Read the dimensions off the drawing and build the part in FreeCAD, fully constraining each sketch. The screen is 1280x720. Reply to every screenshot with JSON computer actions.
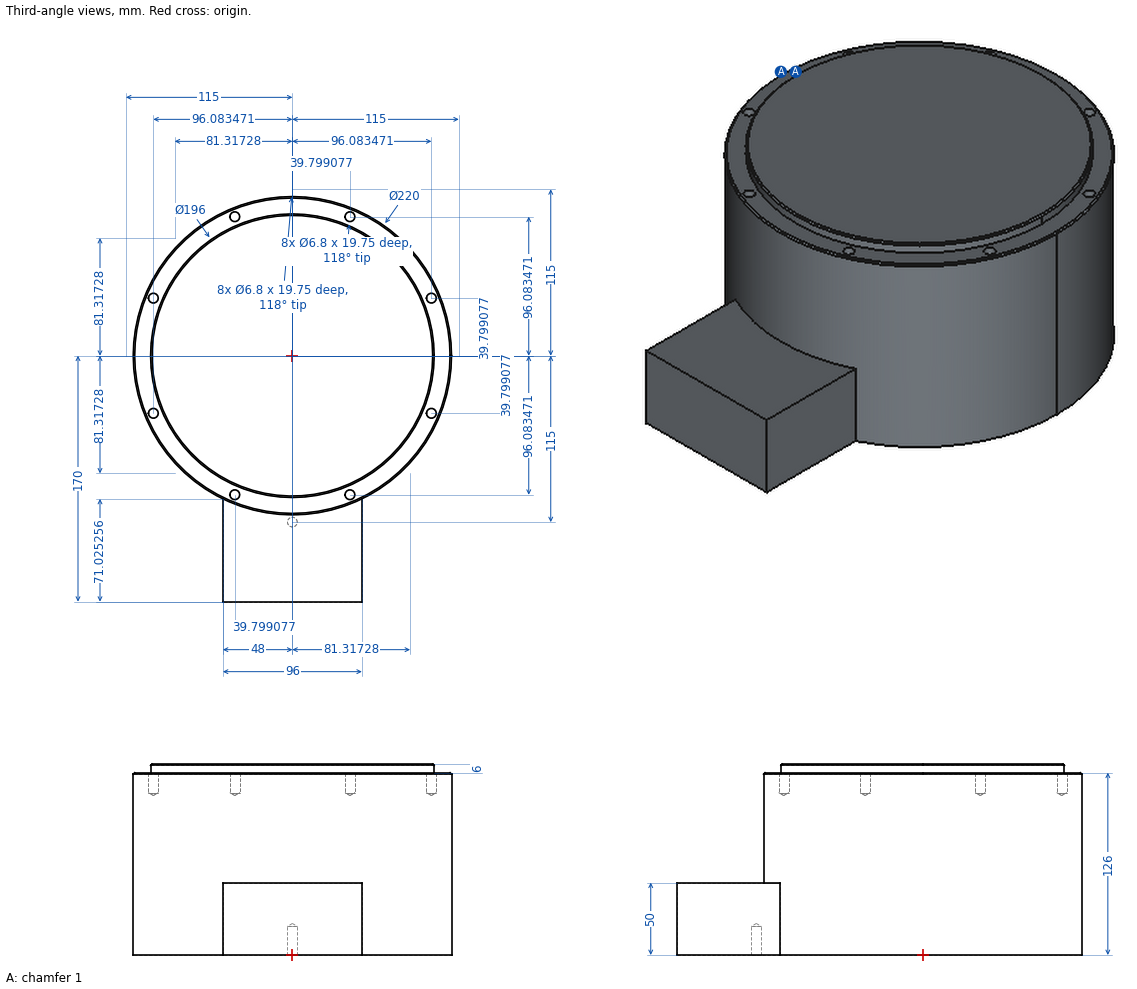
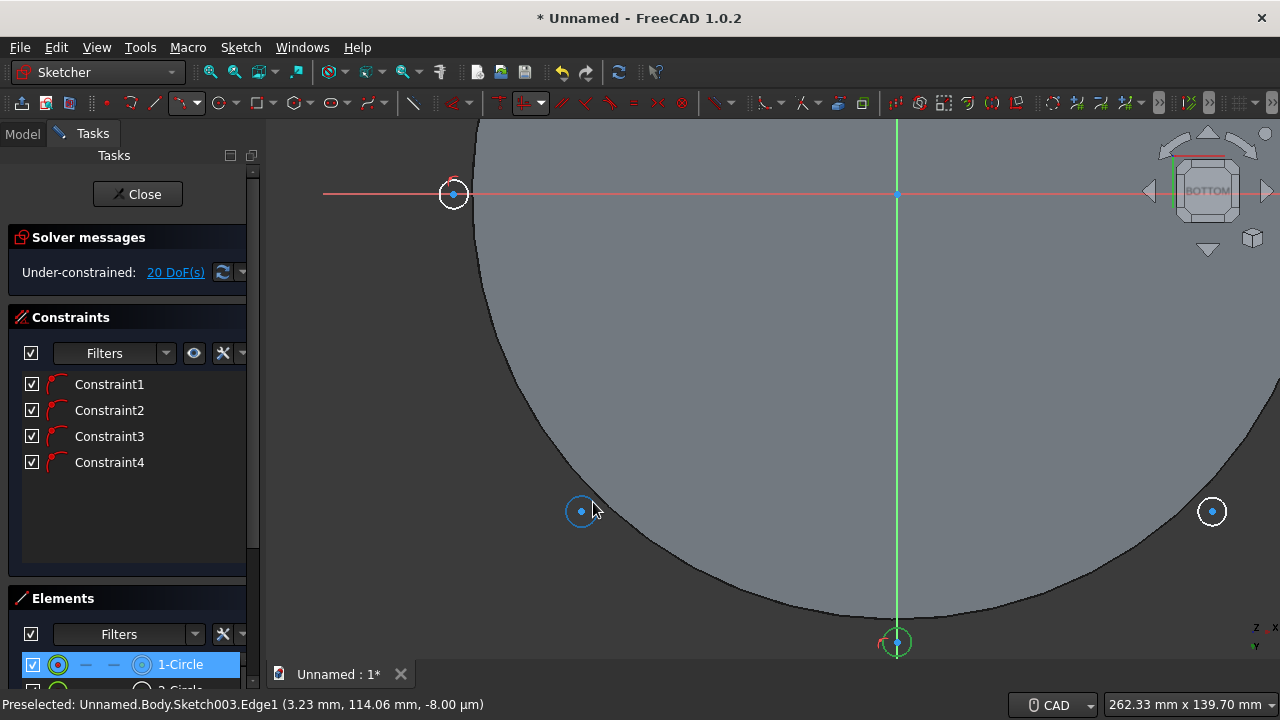
{"action": "left_click", "coordinate": [592, 501]}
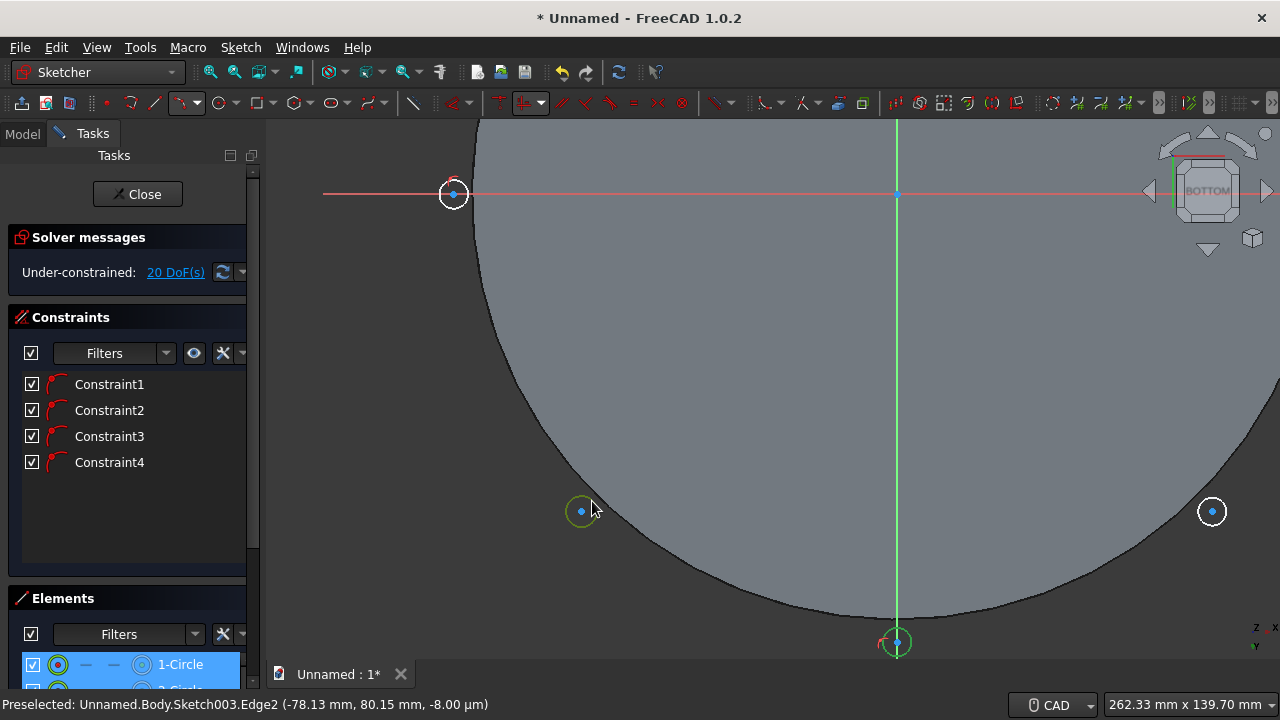
{"action": "scroll", "coordinate": [464, 184], "scroll_direction": "up", "scroll_amount": 2}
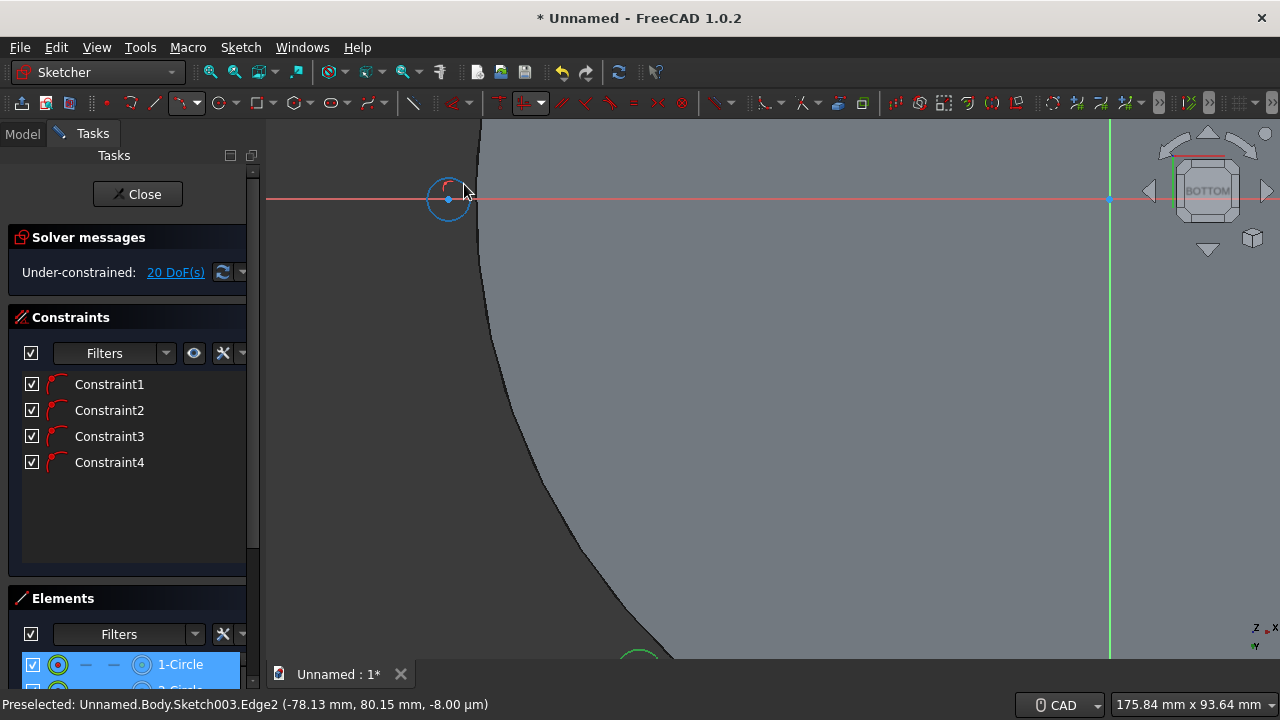
{"action": "left_click", "coordinate": [464, 184]}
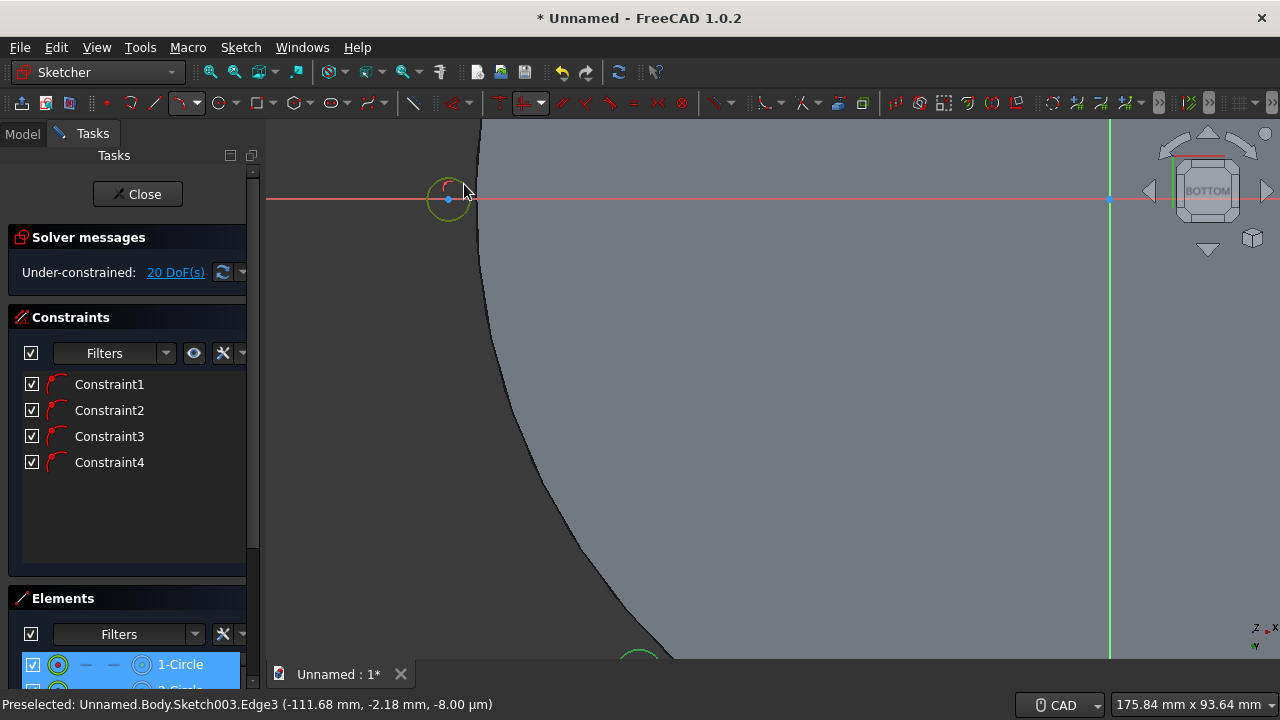
{"action": "scroll", "coordinate": [572, 451], "scroll_direction": "down", "scroll_amount": 7}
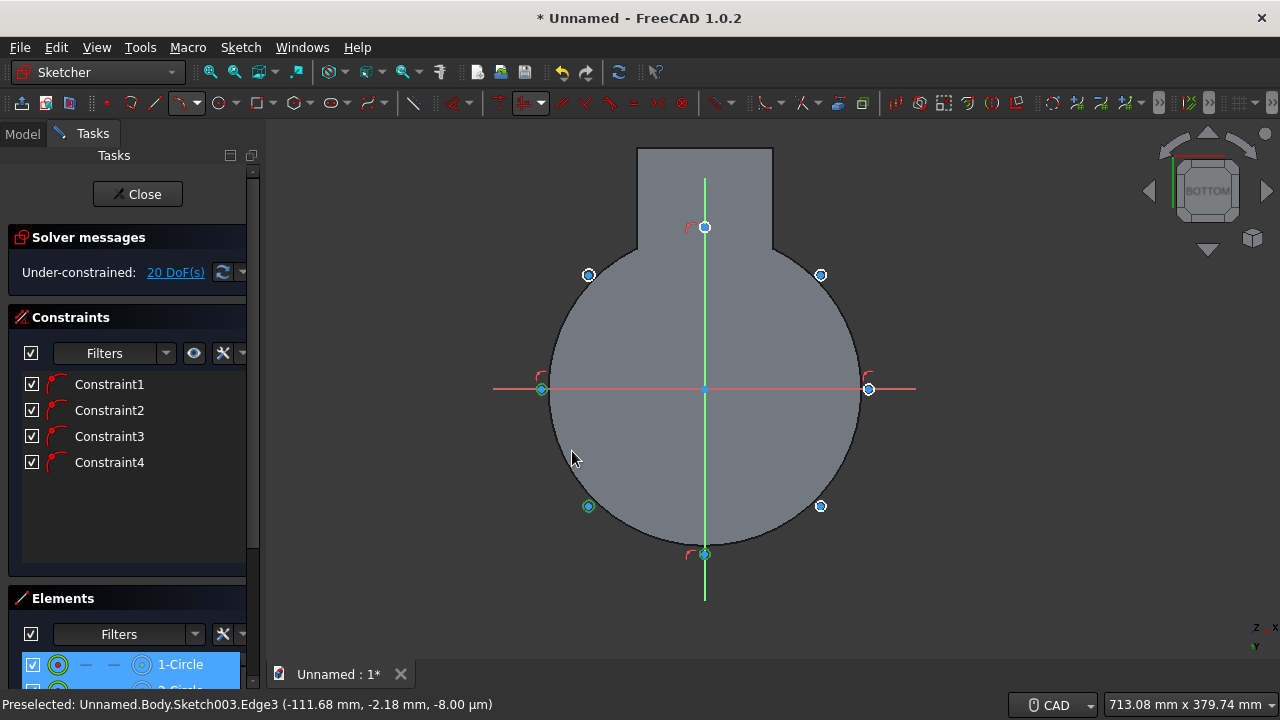
{"action": "scroll", "coordinate": [593, 271], "scroll_direction": "up", "scroll_amount": 5}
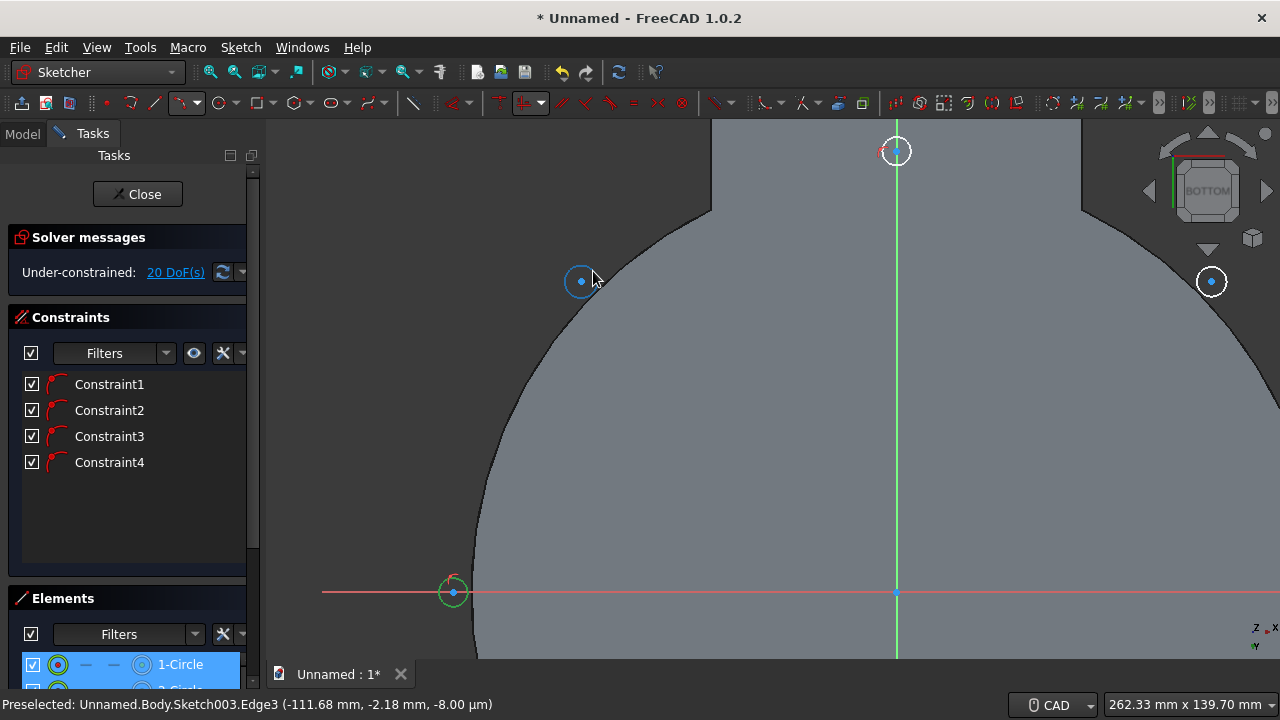
{"action": "left_click", "coordinate": [593, 270]}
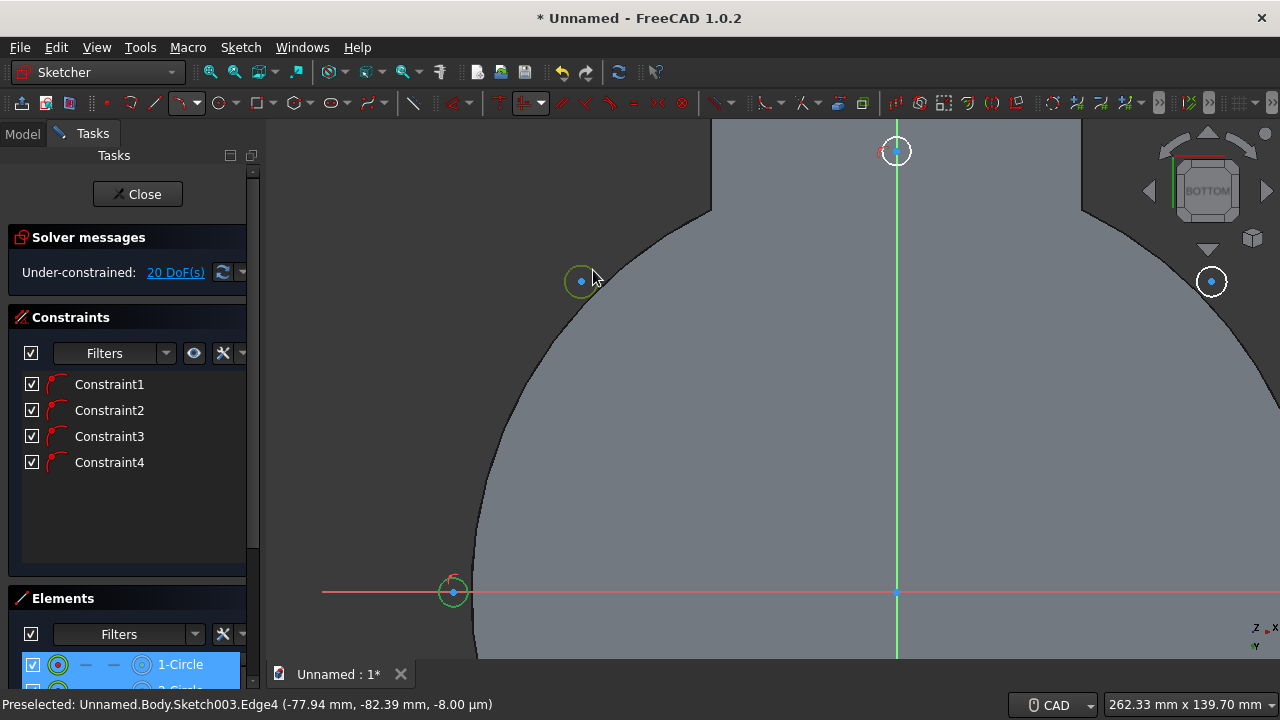
{"action": "scroll", "coordinate": [887, 161], "scroll_direction": "up", "scroll_amount": 2}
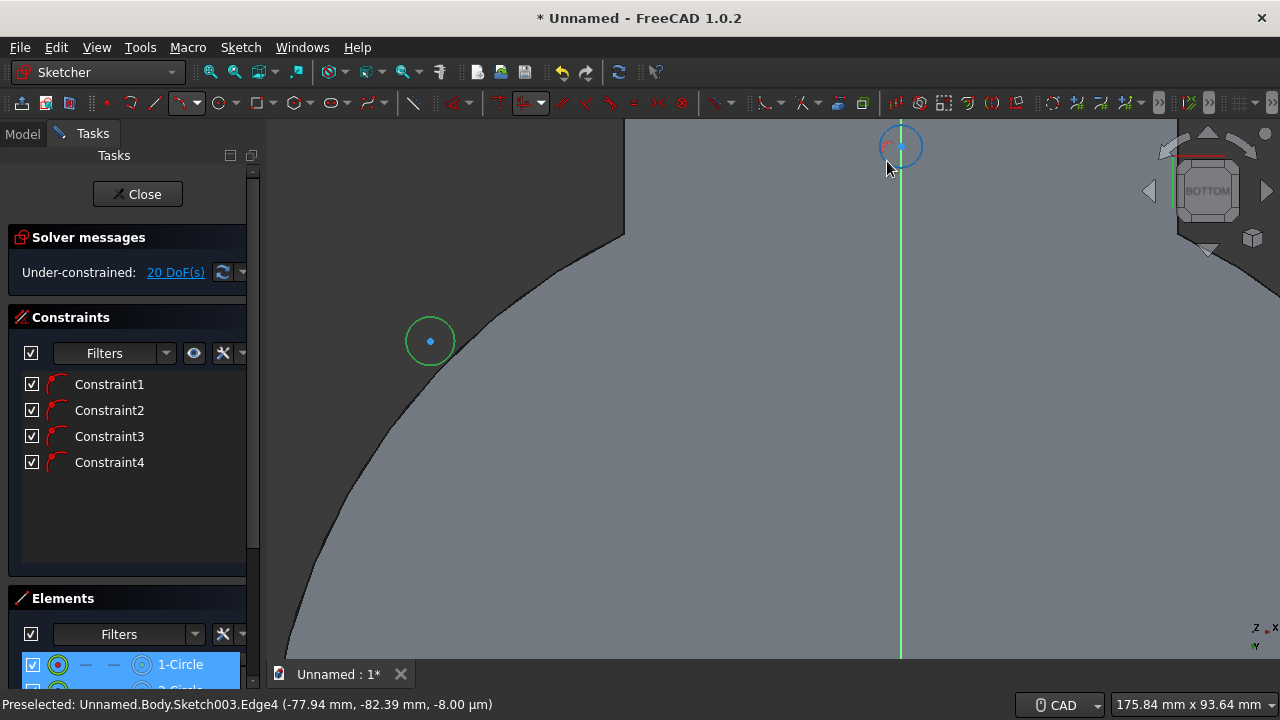
{"action": "left_click", "coordinate": [886, 161]}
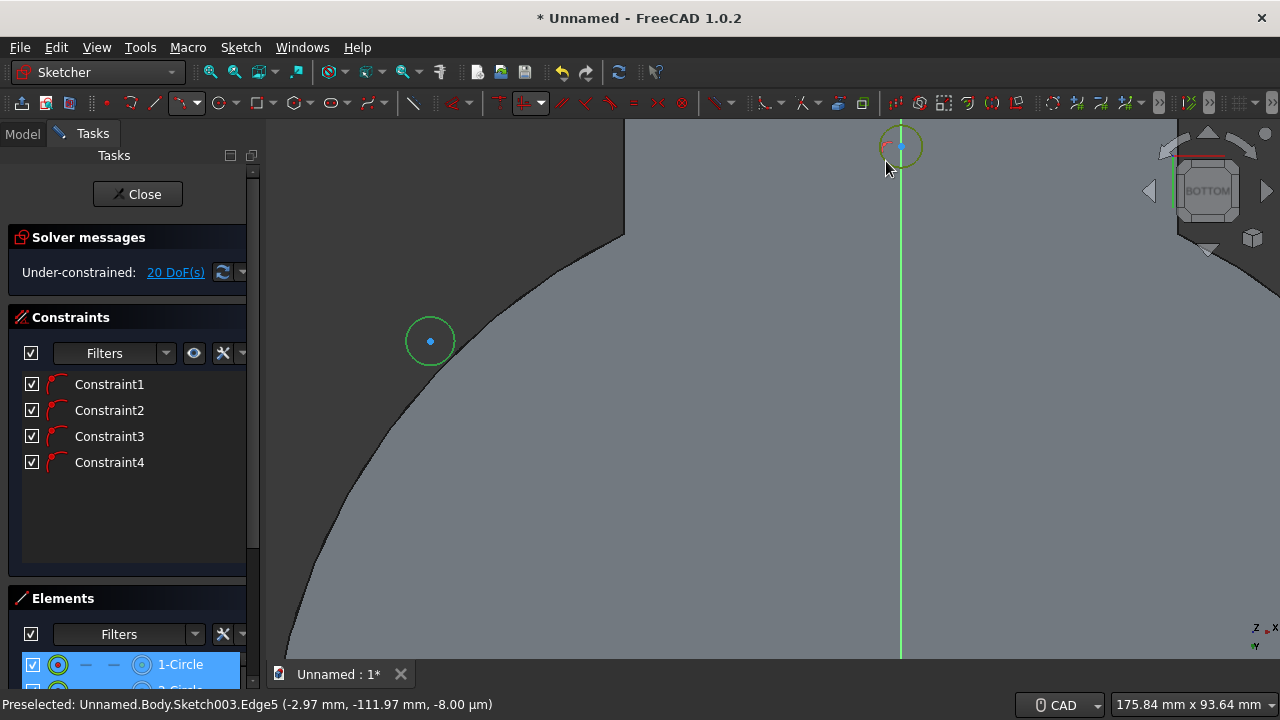
{"action": "scroll", "coordinate": [640, 253], "scroll_direction": "down", "scroll_amount": 7}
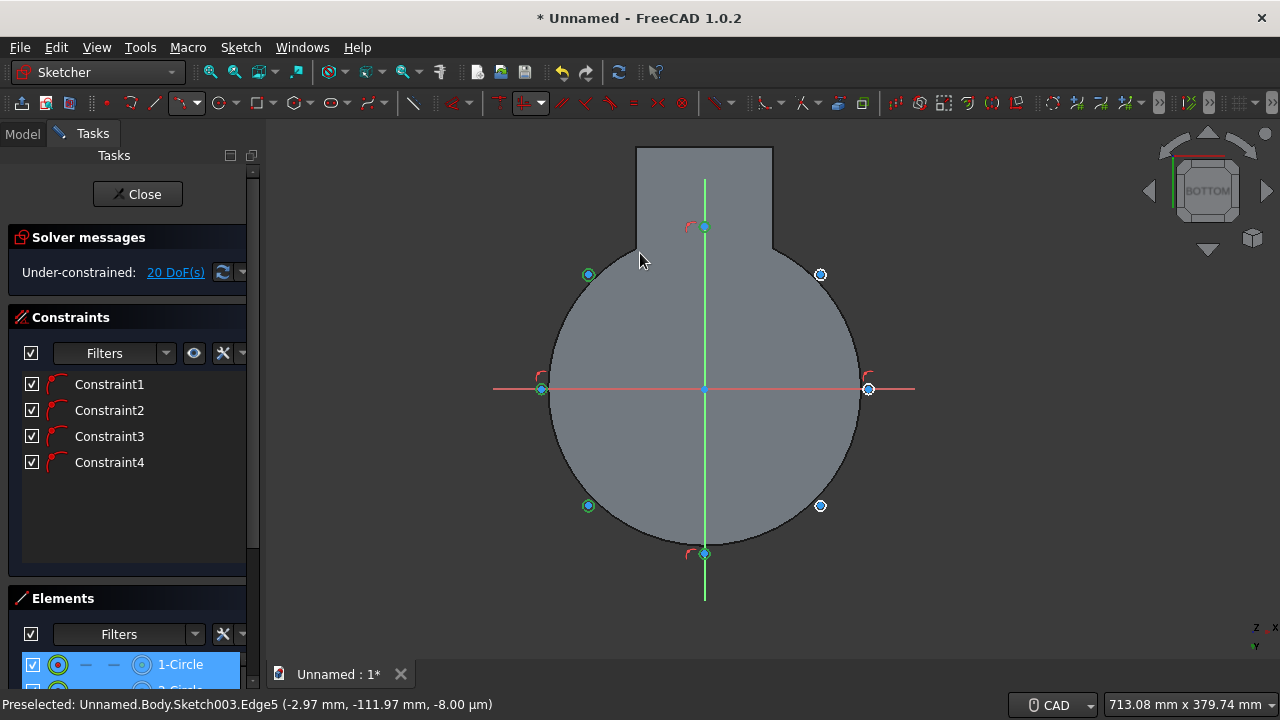
{"action": "scroll", "coordinate": [824, 271], "scroll_direction": "up", "scroll_amount": 5}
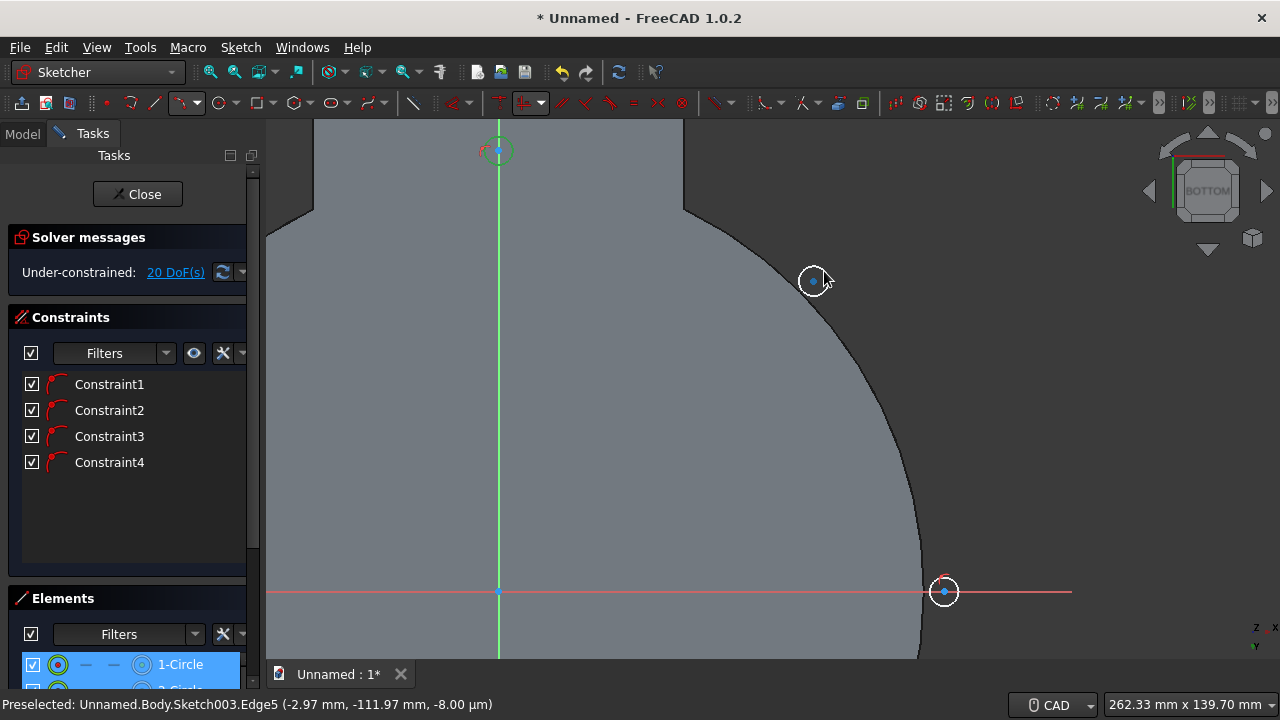
{"action": "left_click", "coordinate": [824, 271]}